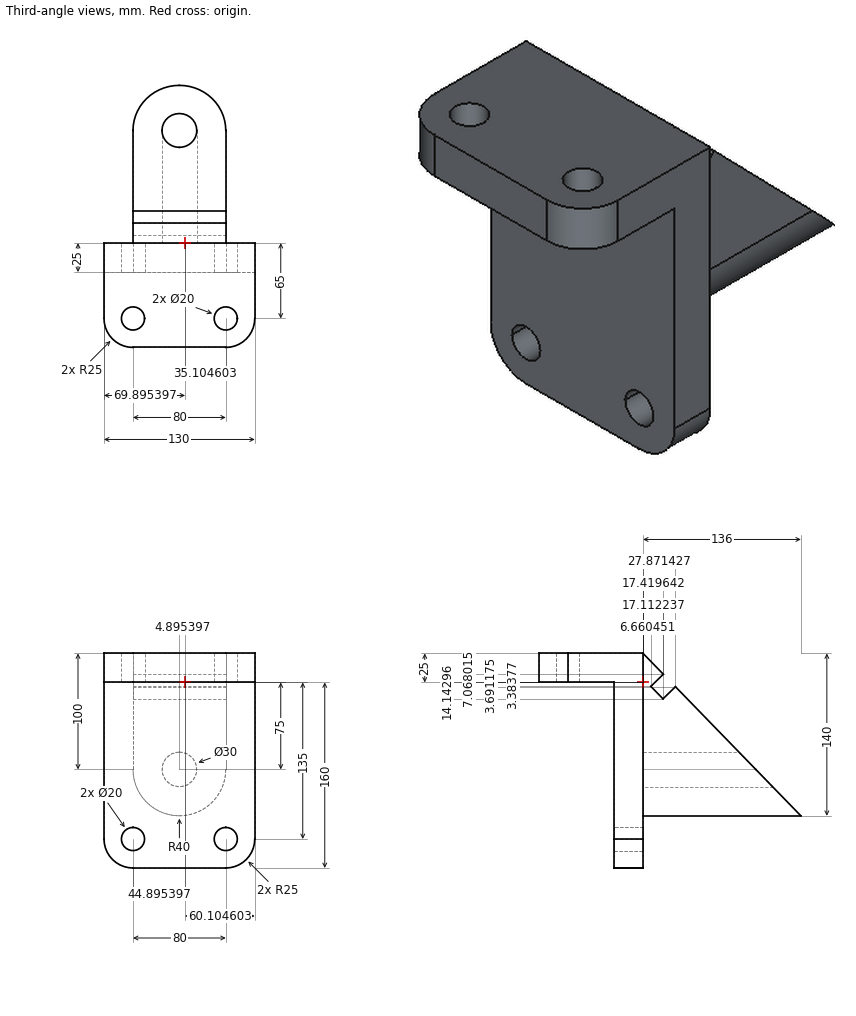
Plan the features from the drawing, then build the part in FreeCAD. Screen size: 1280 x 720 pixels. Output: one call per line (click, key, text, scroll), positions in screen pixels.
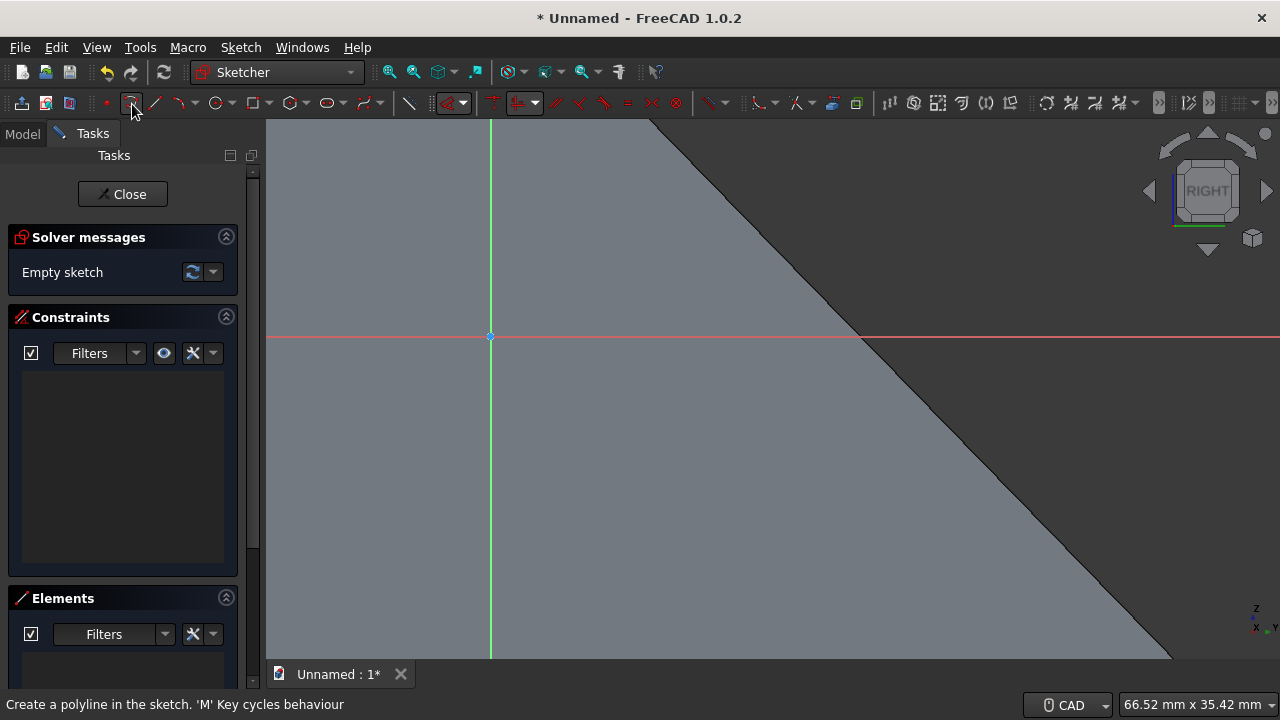
click(592, 388)
click(752, 552)
click(916, 393)
click(756, 229)
click(592, 389)
key(Escape)
key(Escape)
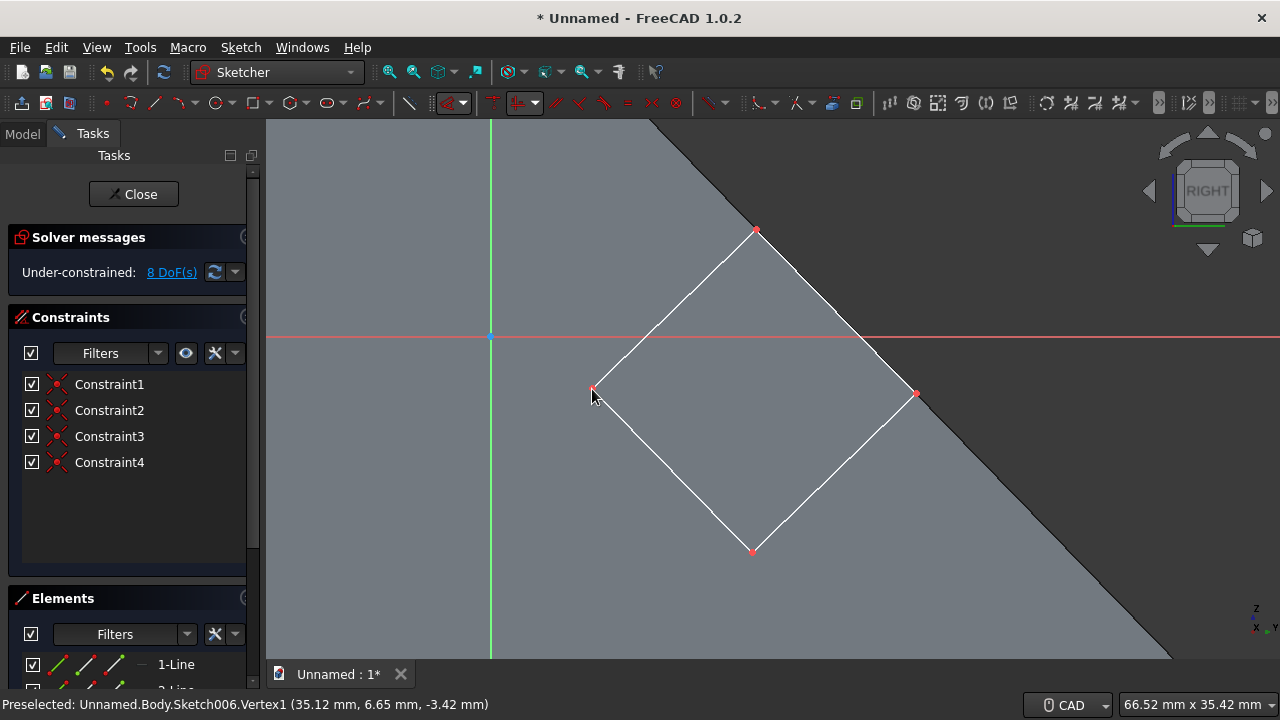
click(592, 389)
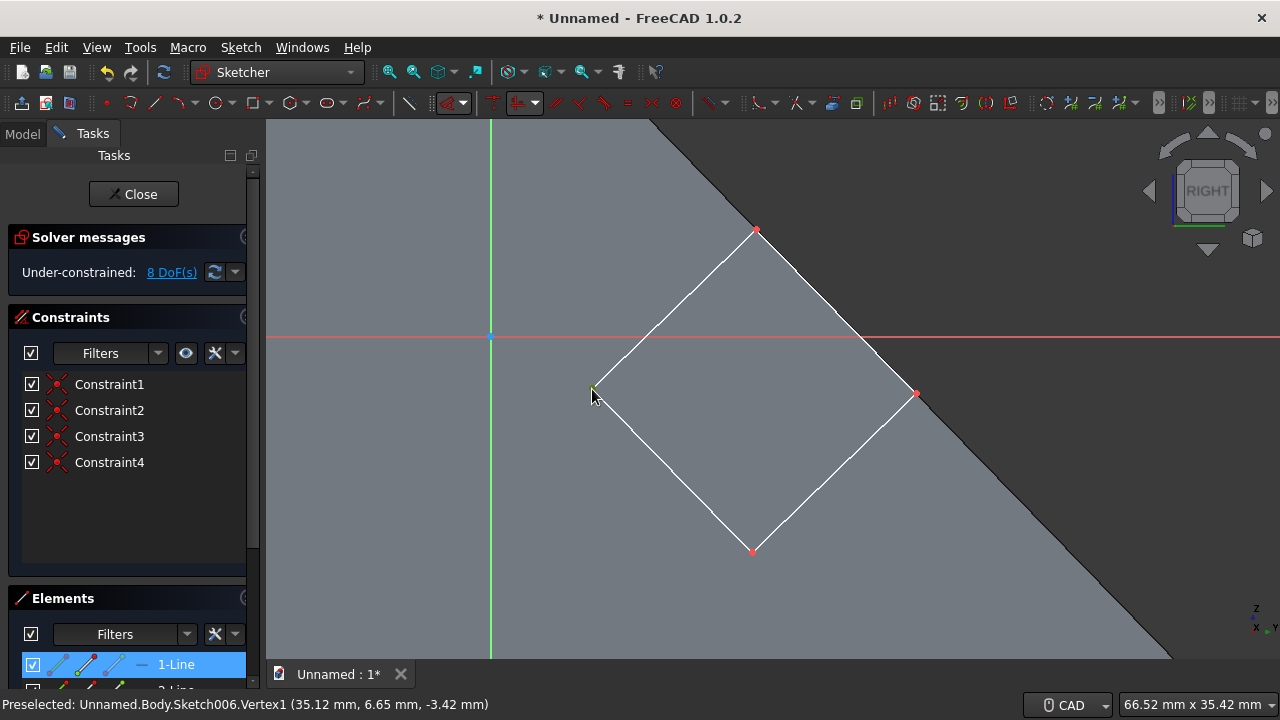
key(i)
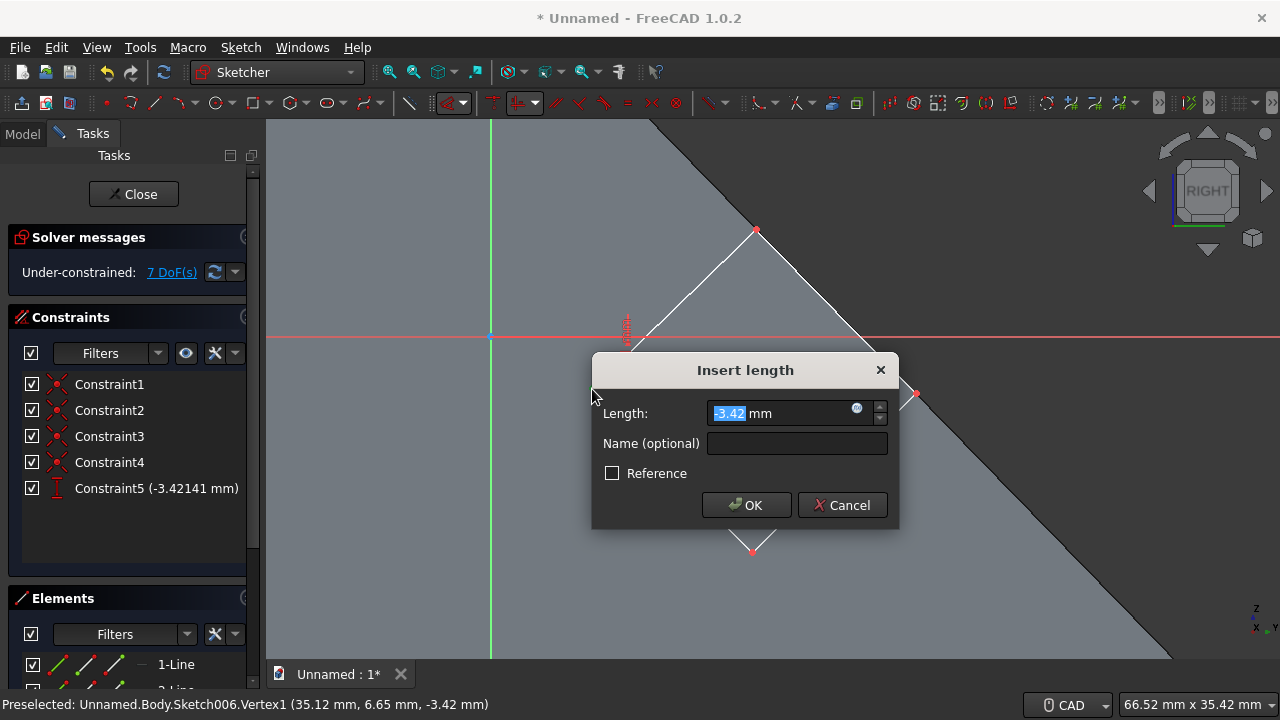
text(-3.38377)
key(Return)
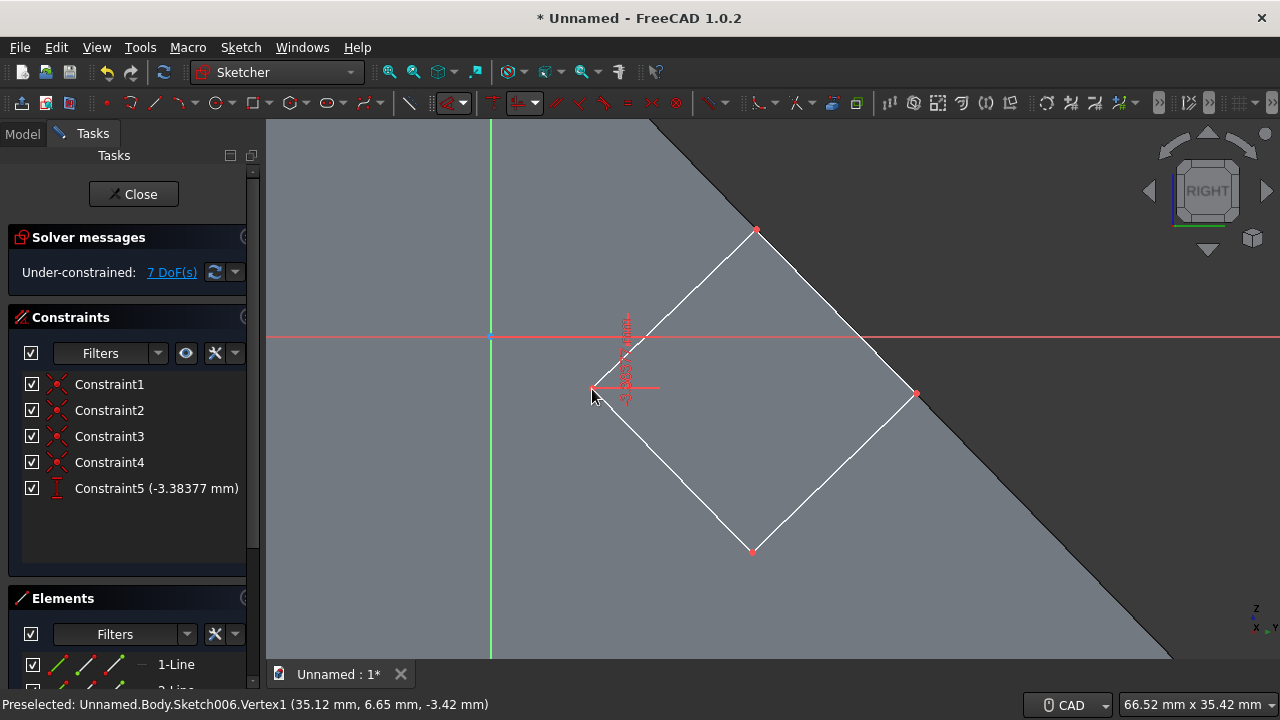
click(592, 388)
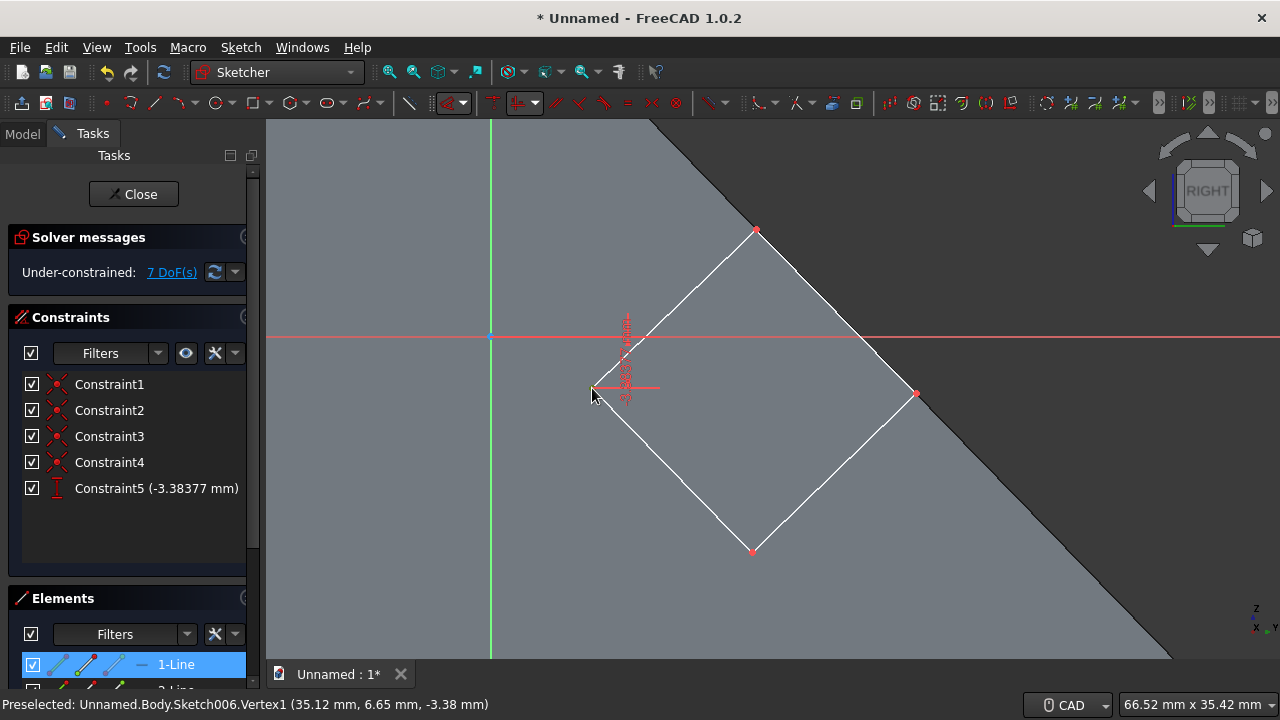
click(466, 104)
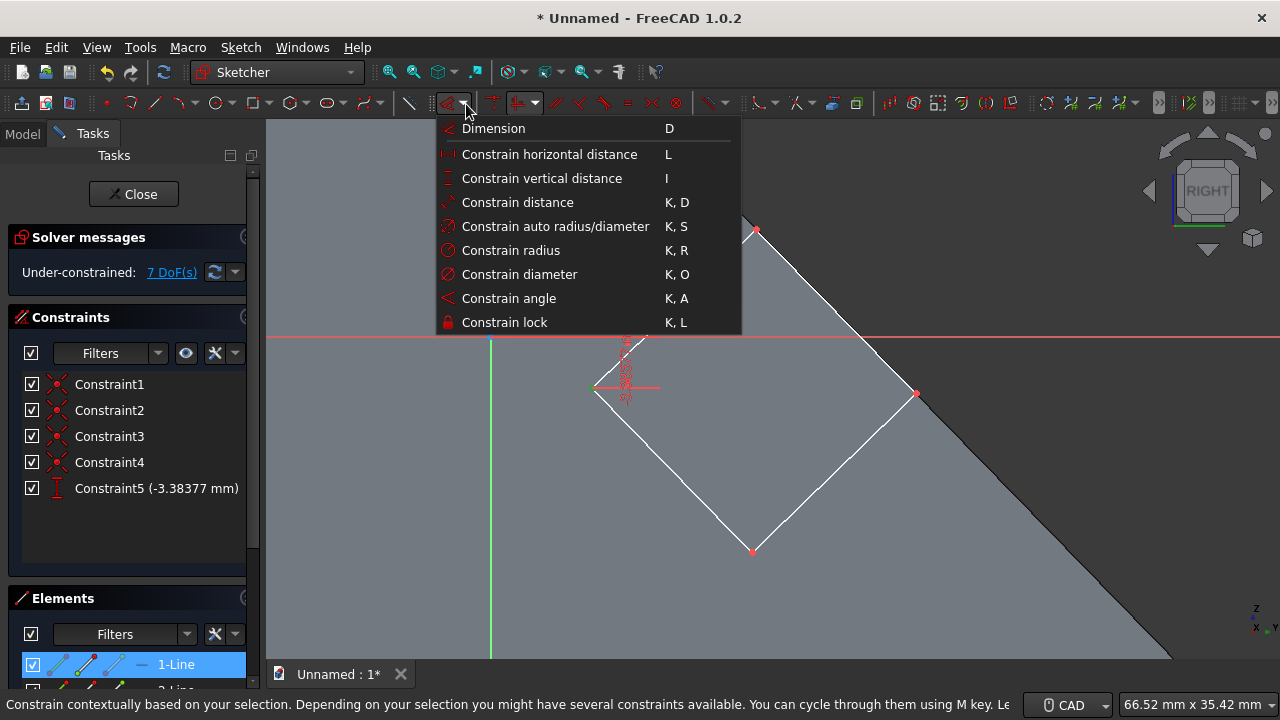
click(589, 154)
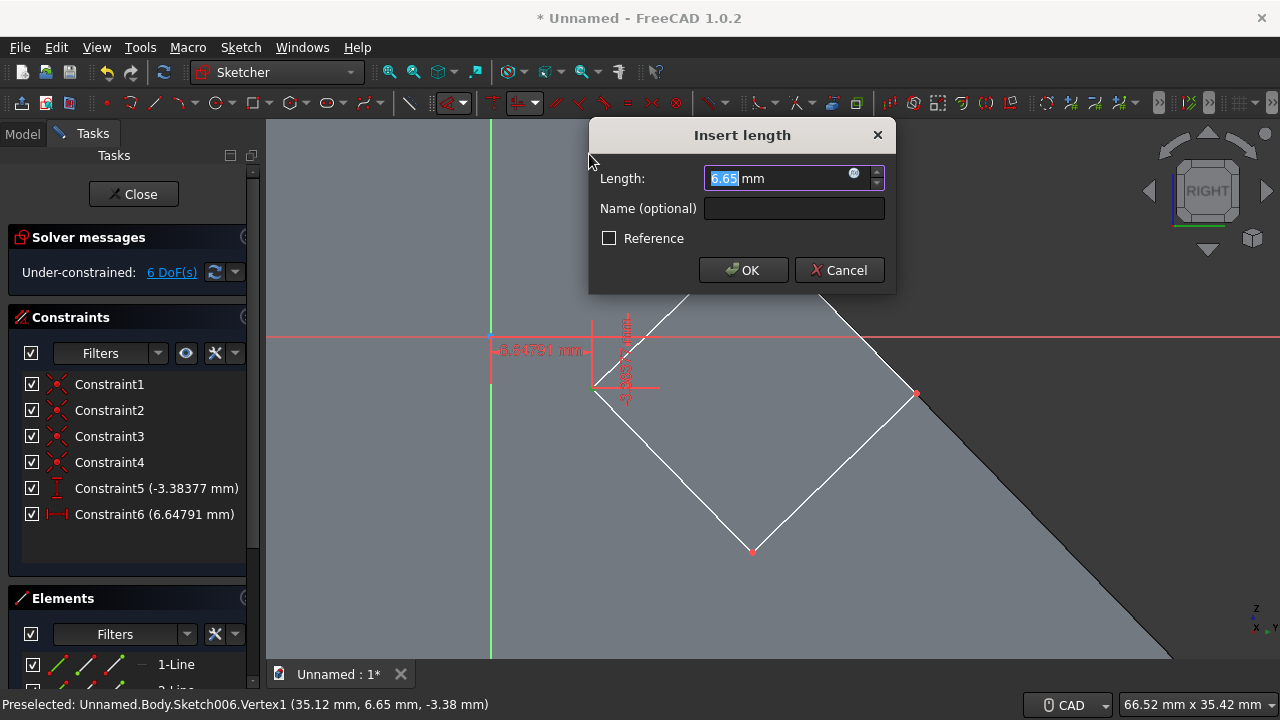
text(6.660451)
key(Return)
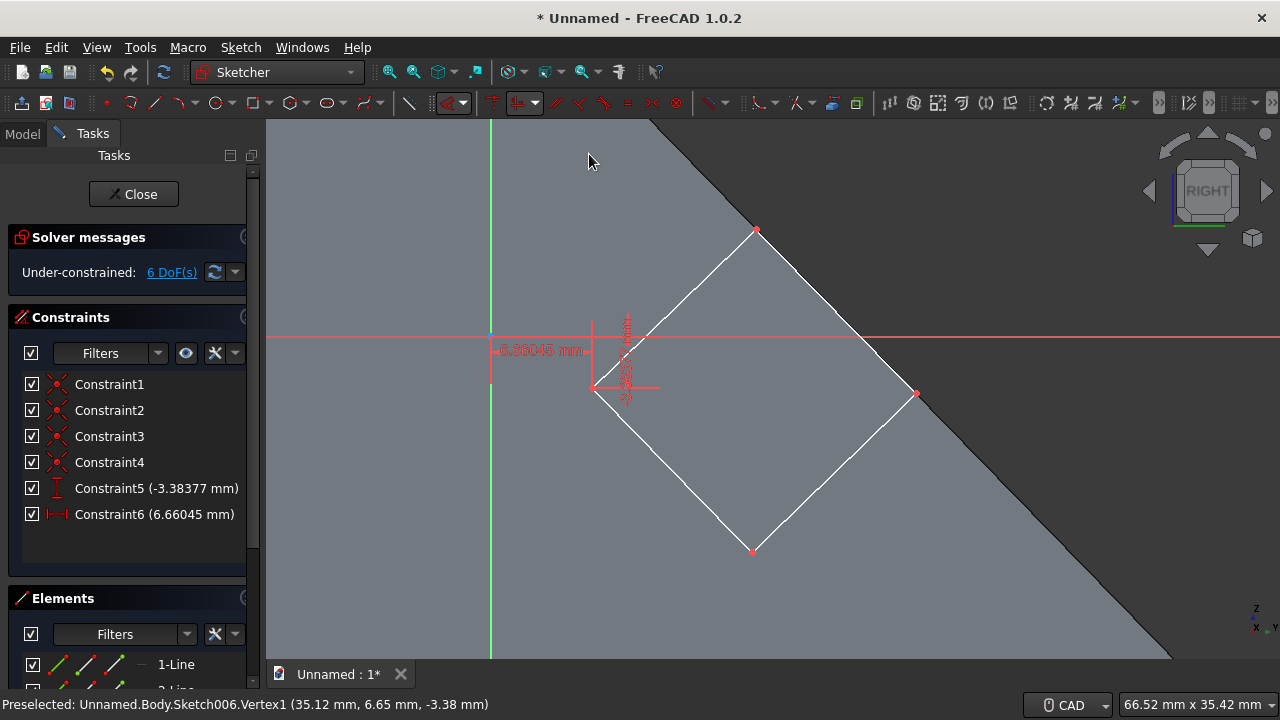
click(752, 553)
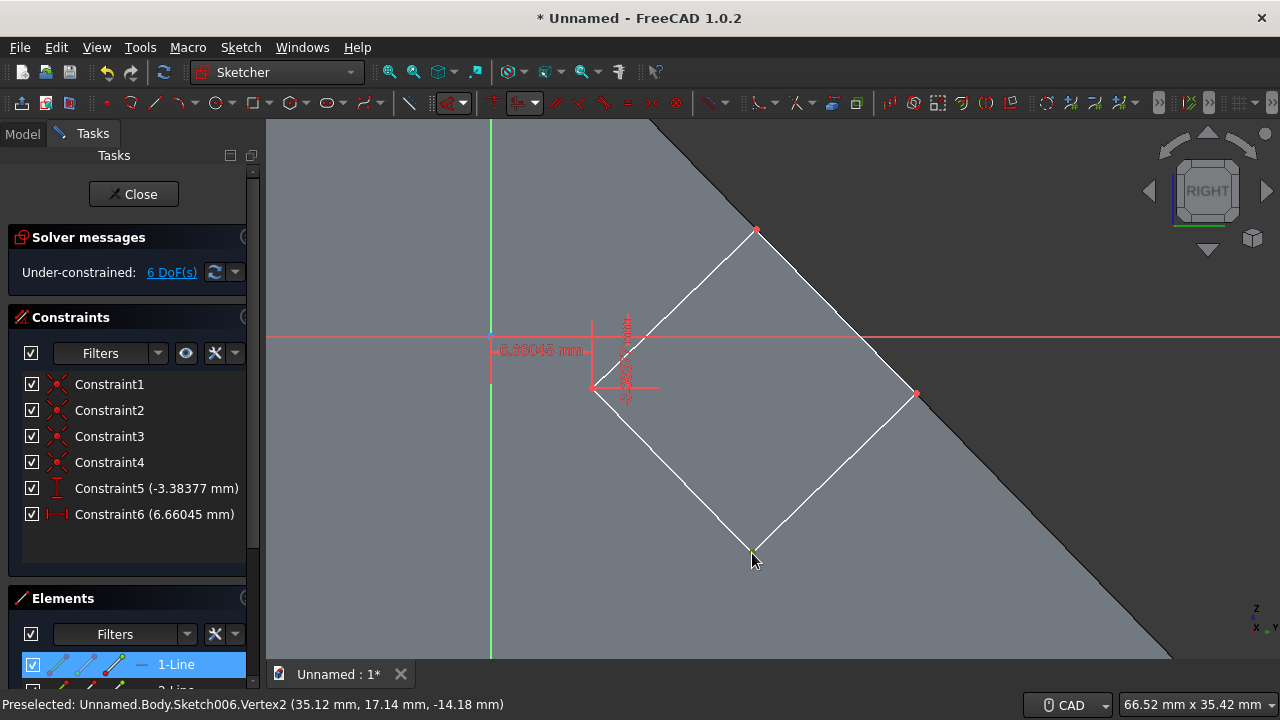
key(i)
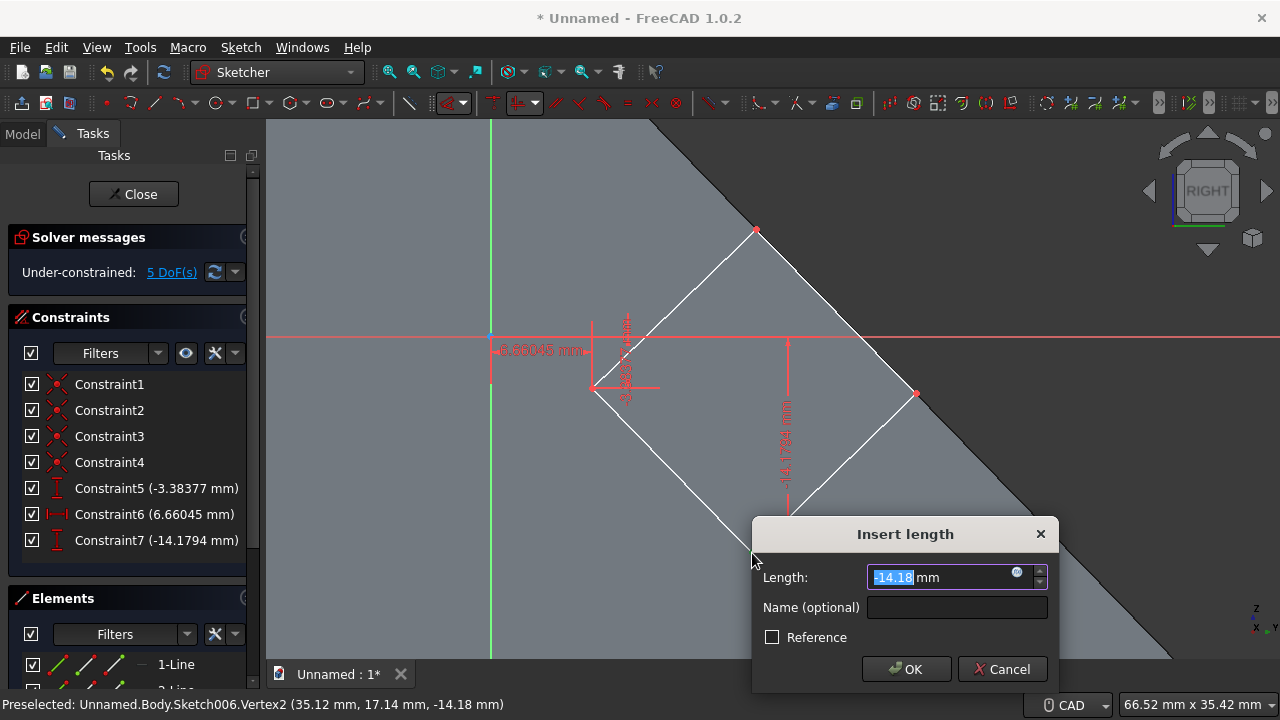
text(-14.14296)
key(Return)